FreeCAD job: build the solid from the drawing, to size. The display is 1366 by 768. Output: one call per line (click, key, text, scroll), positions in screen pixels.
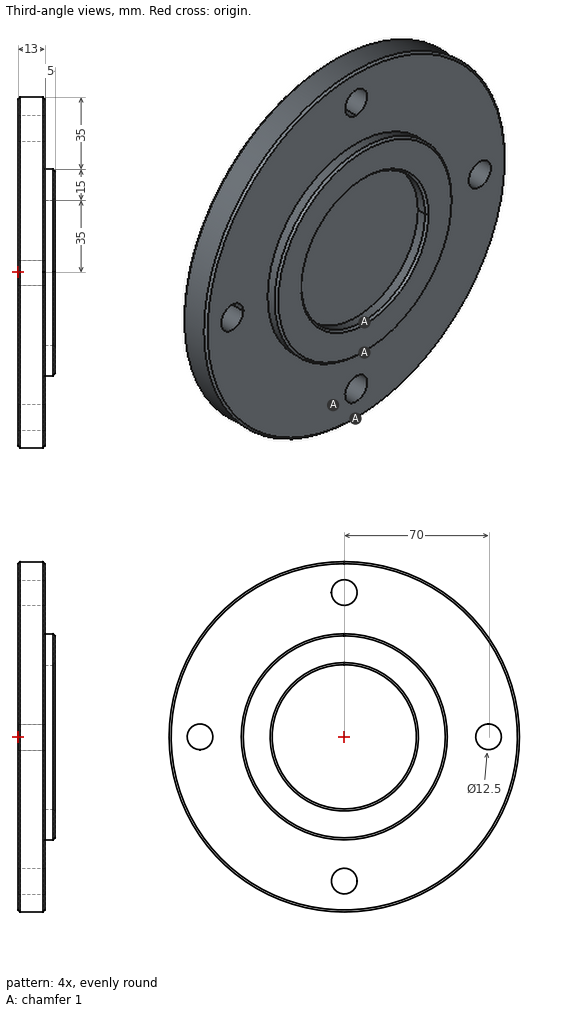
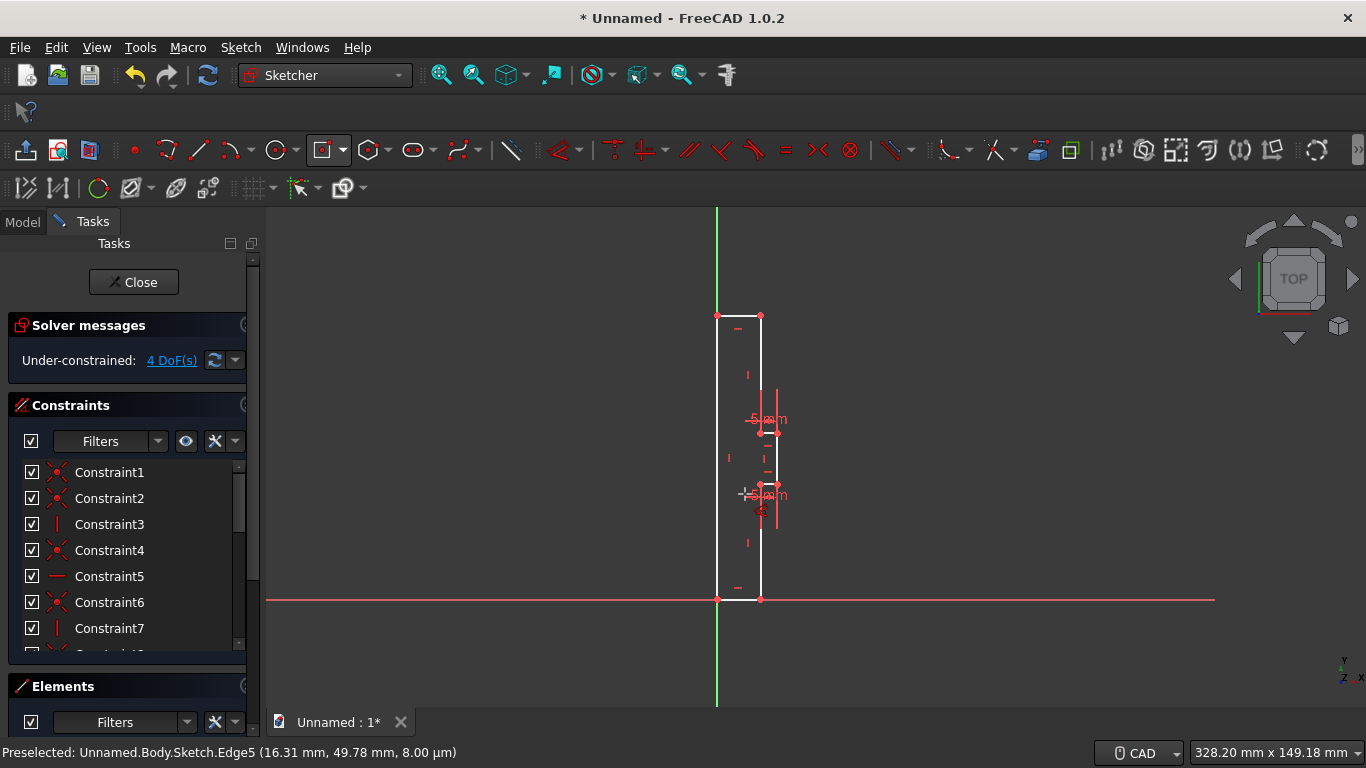
click(730, 600)
click(739, 634)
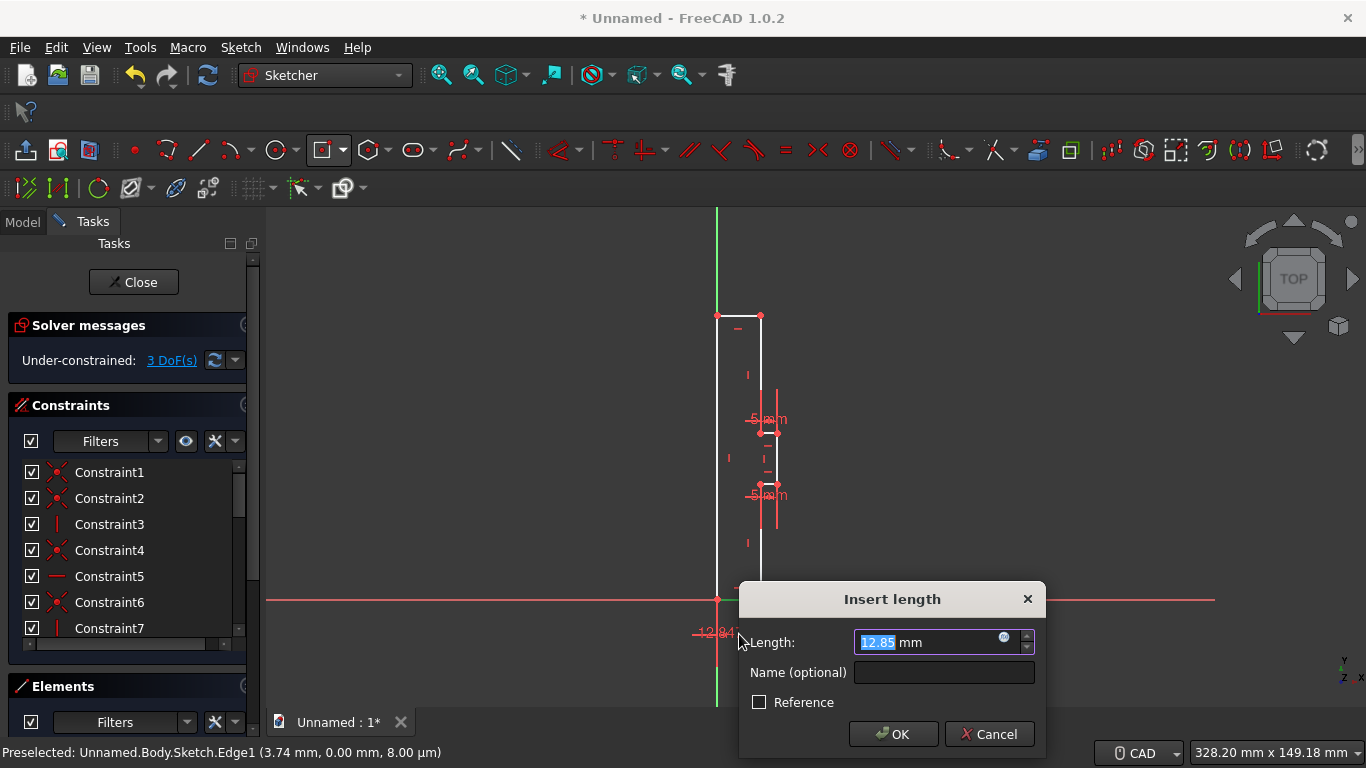
text(13)
key(Return)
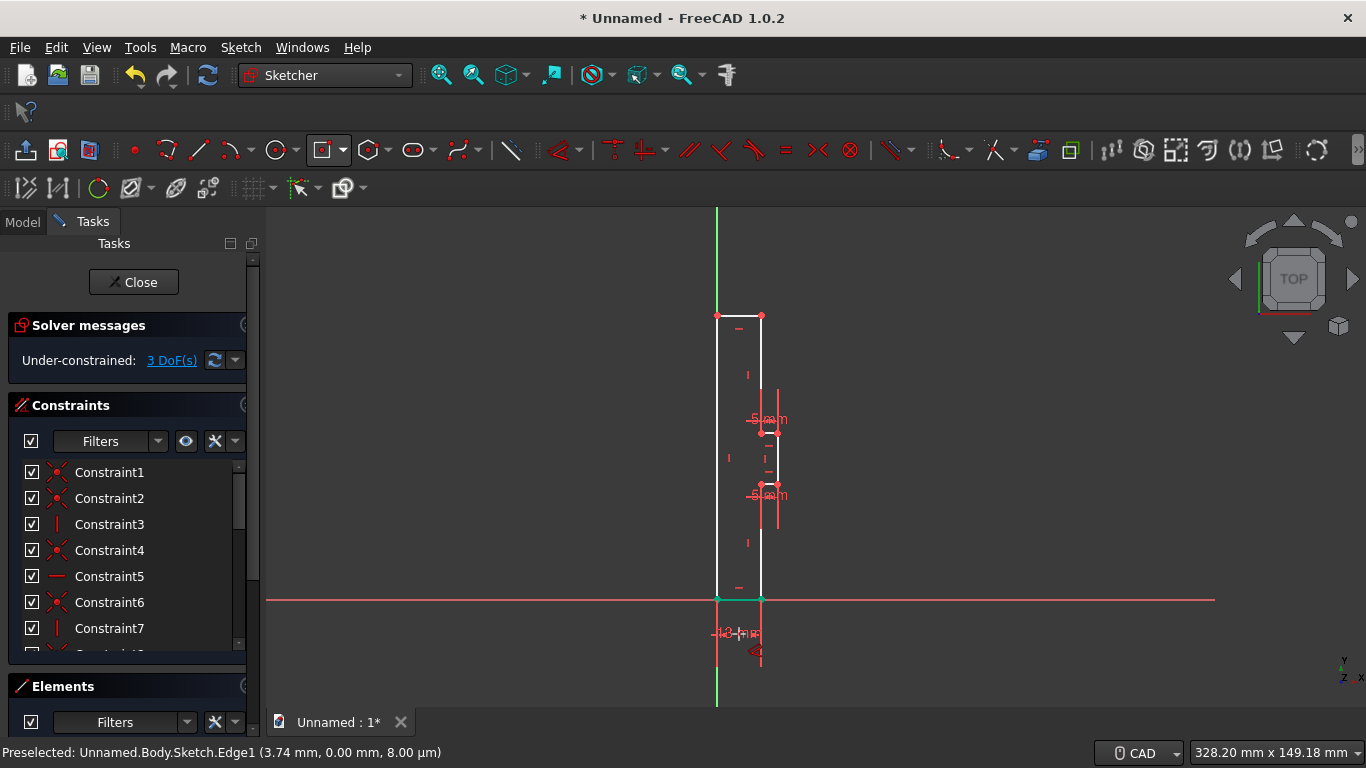
click(761, 565)
click(795, 542)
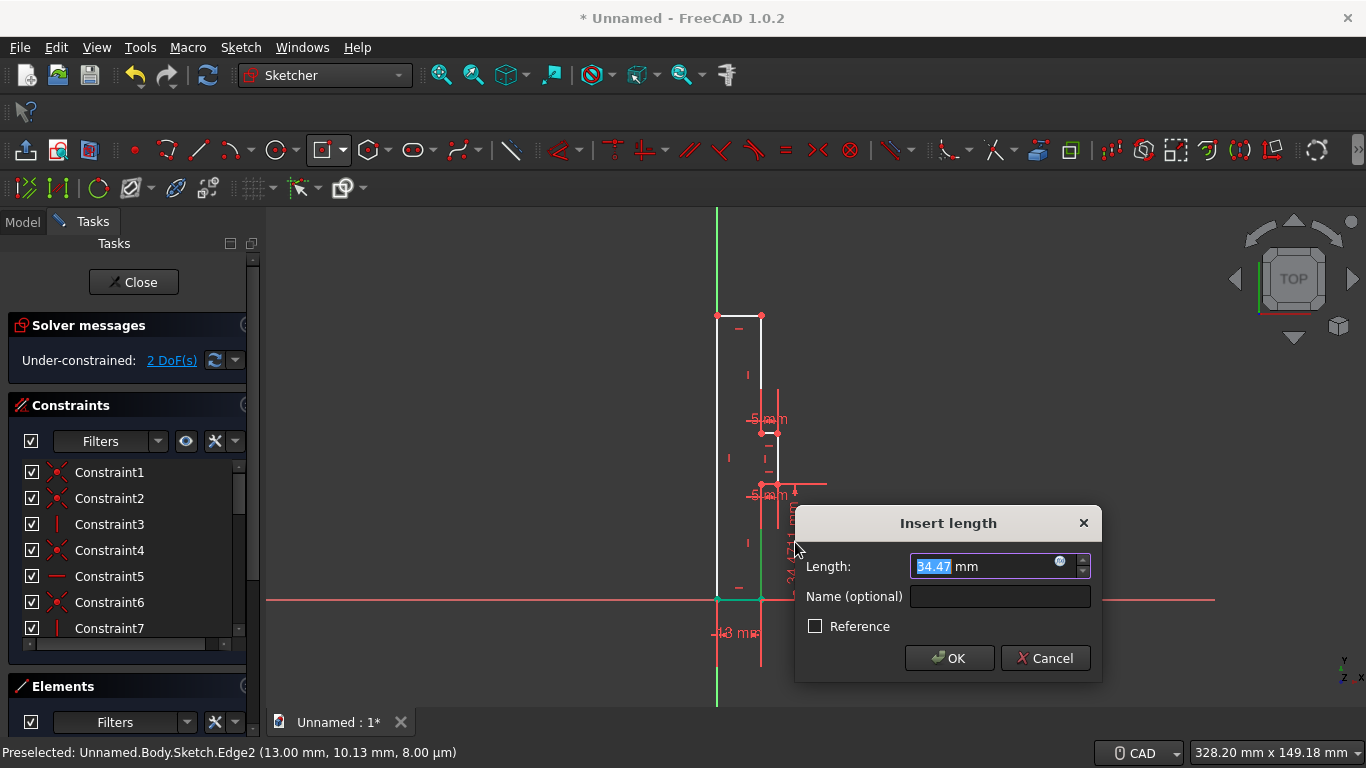
text(35)
key(Return)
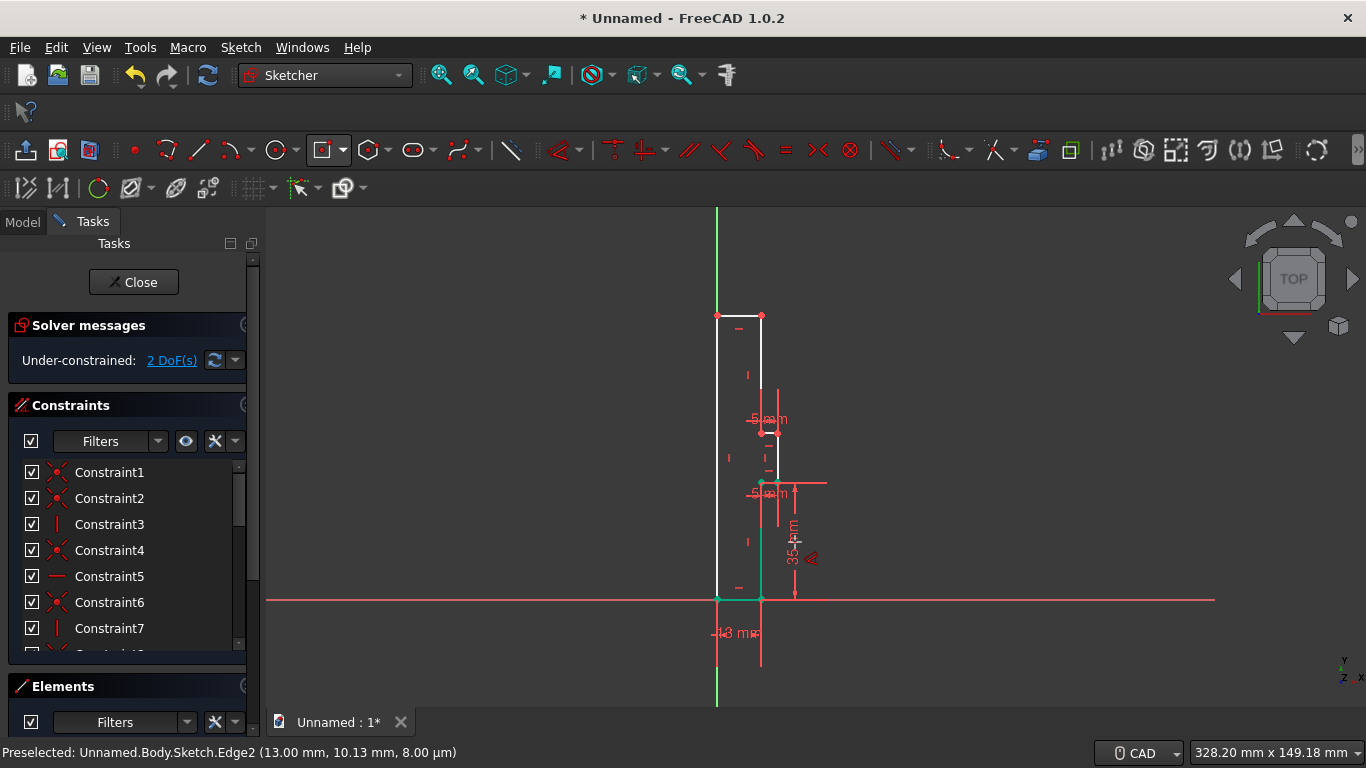
click(778, 468)
click(812, 458)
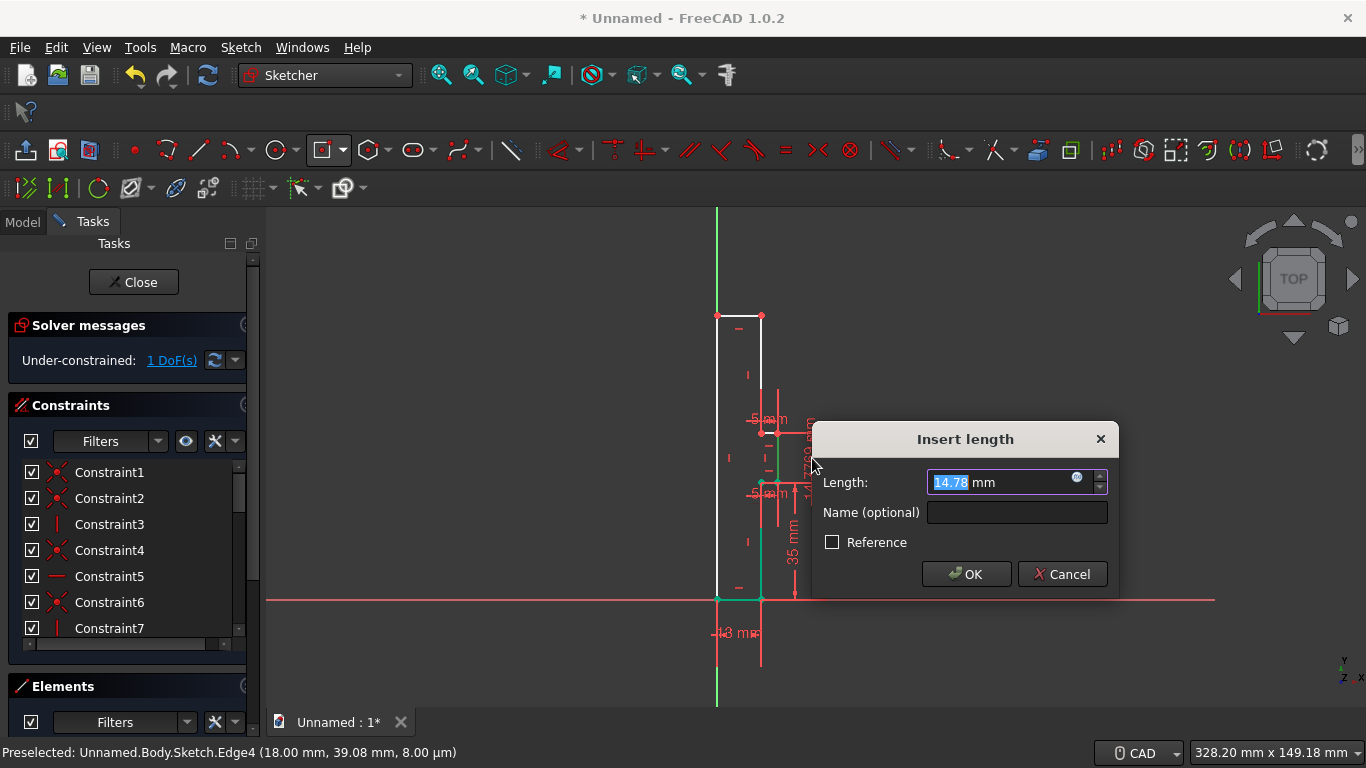
text(15)
key(Return)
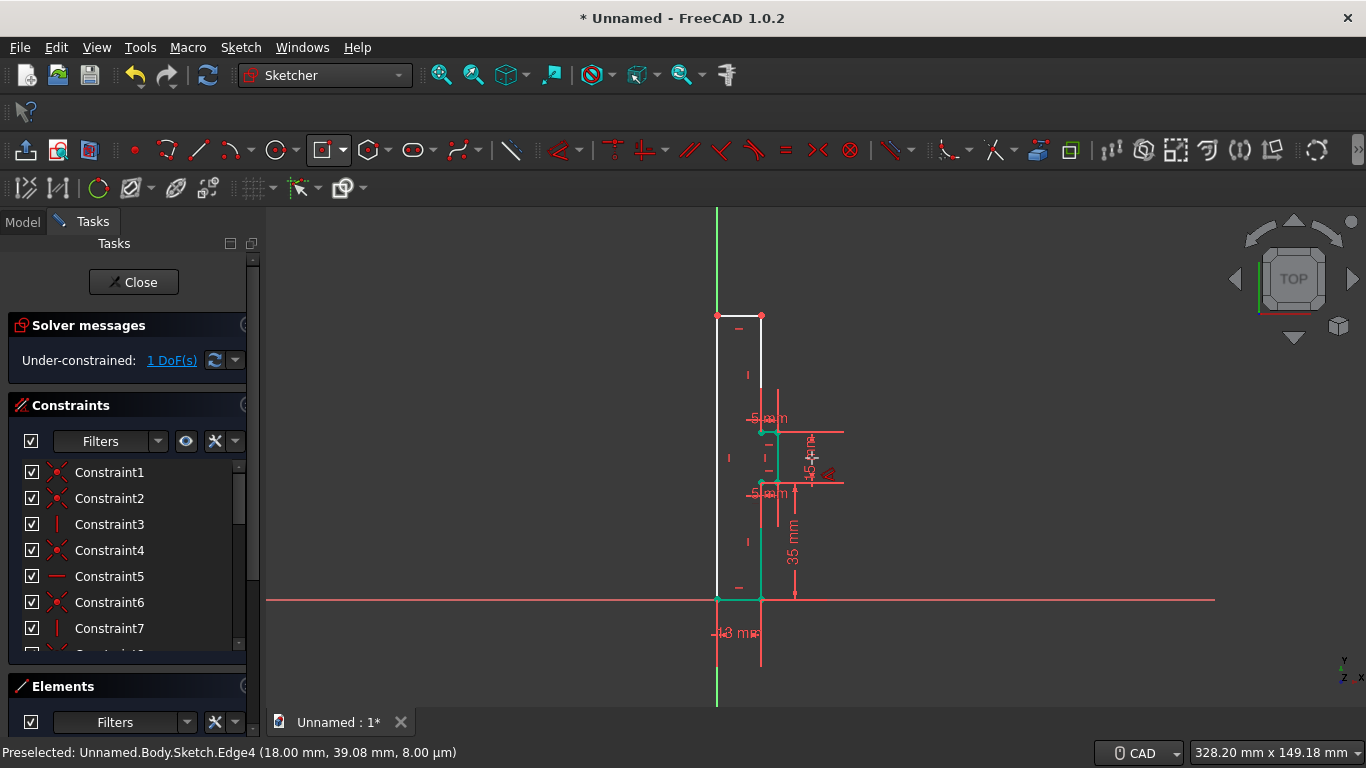
click(761, 397)
click(795, 374)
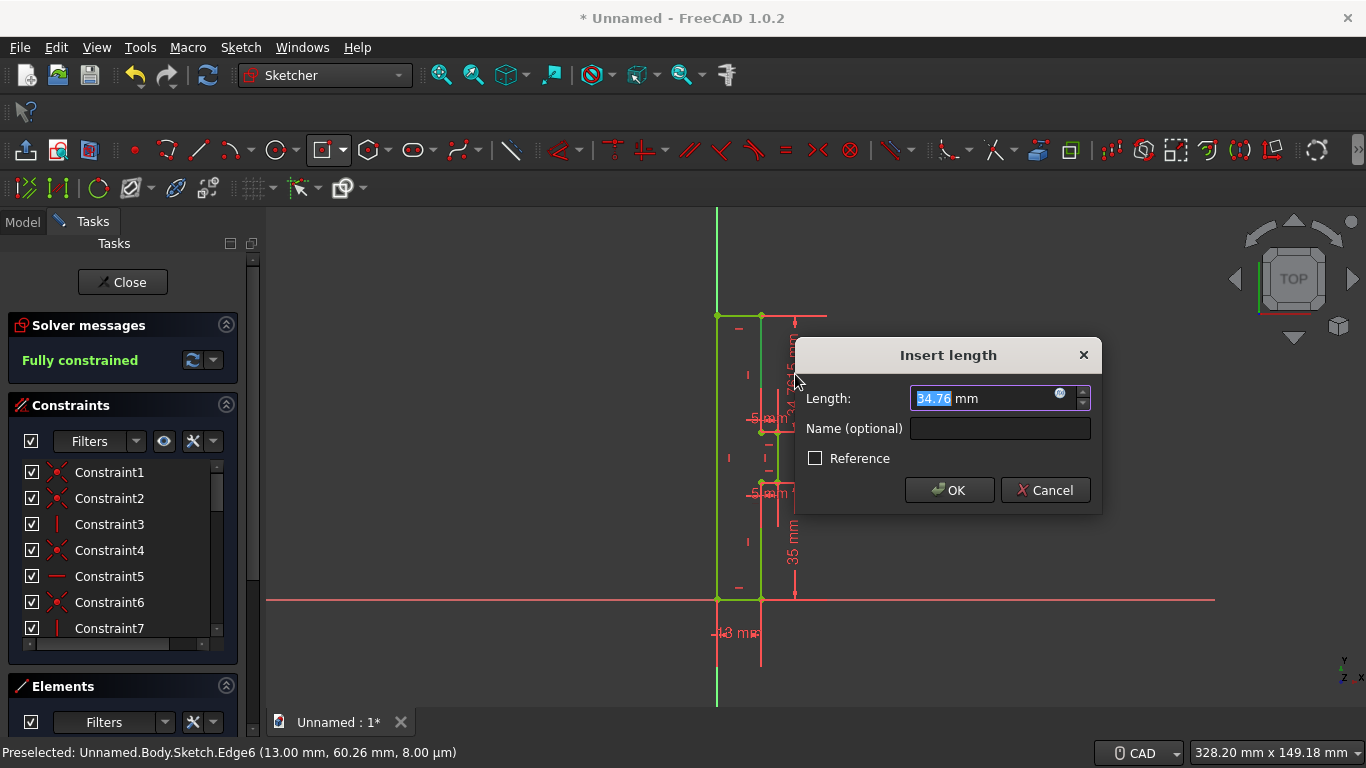
text(35)
key(Return)
key(Escape)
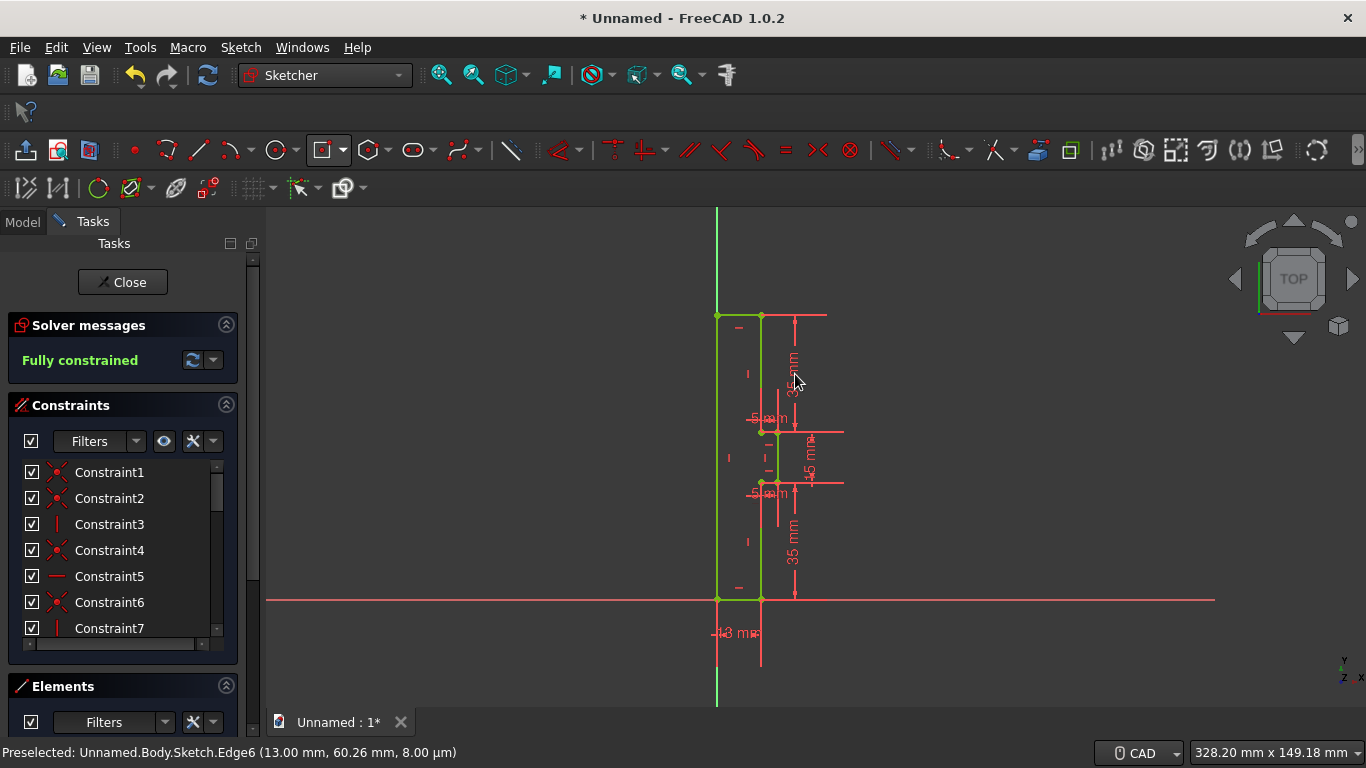
click(123, 282)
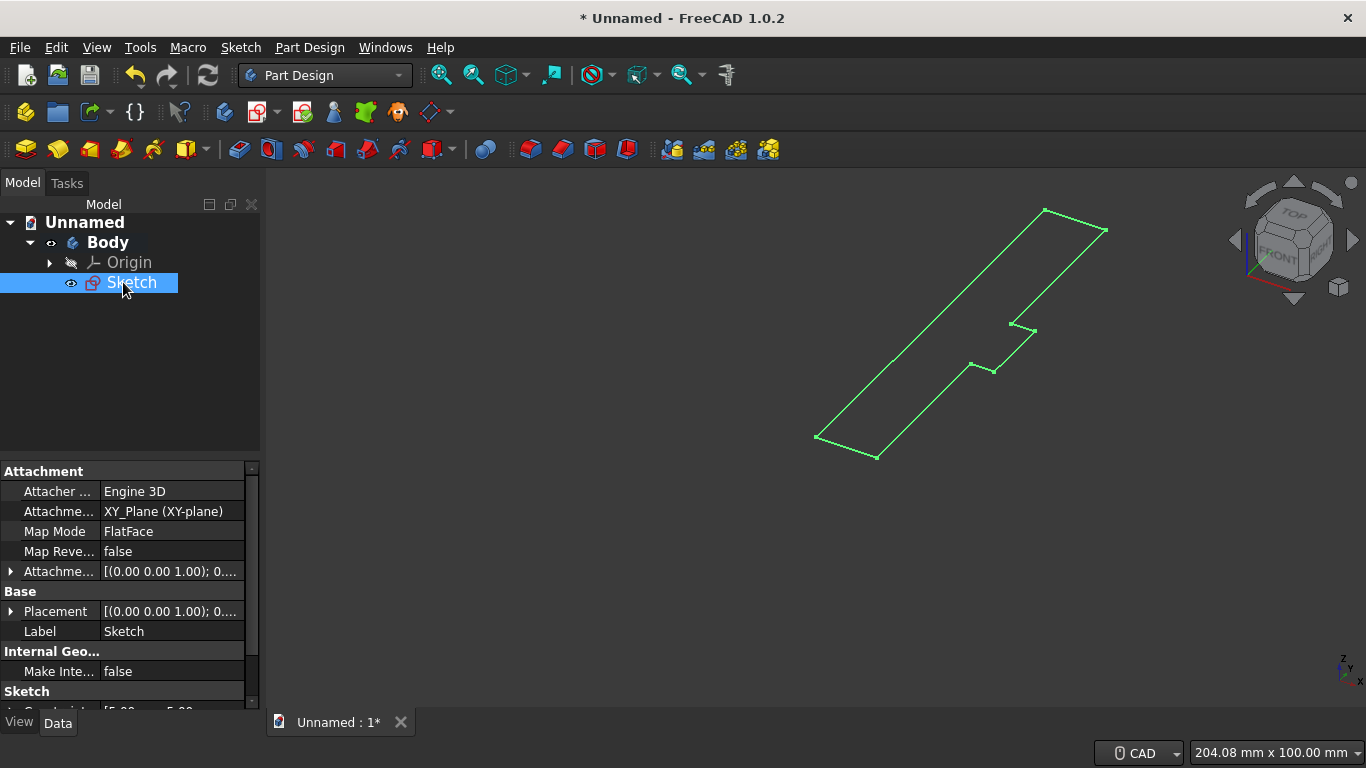
click(58, 150)